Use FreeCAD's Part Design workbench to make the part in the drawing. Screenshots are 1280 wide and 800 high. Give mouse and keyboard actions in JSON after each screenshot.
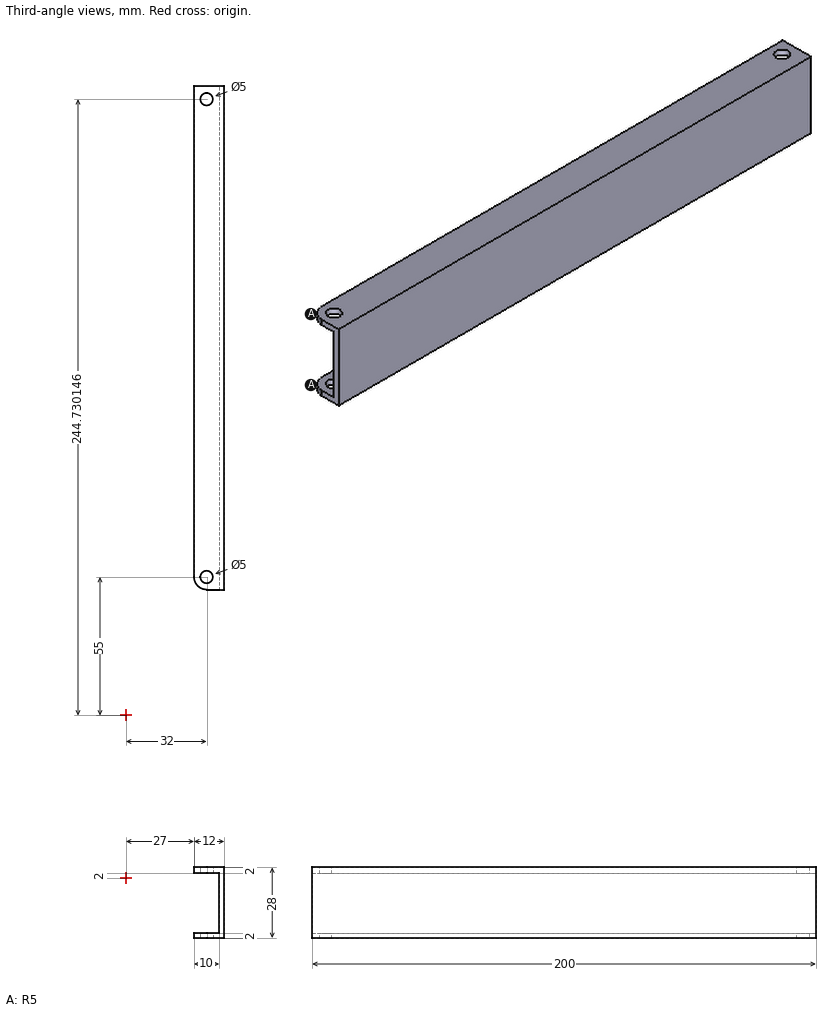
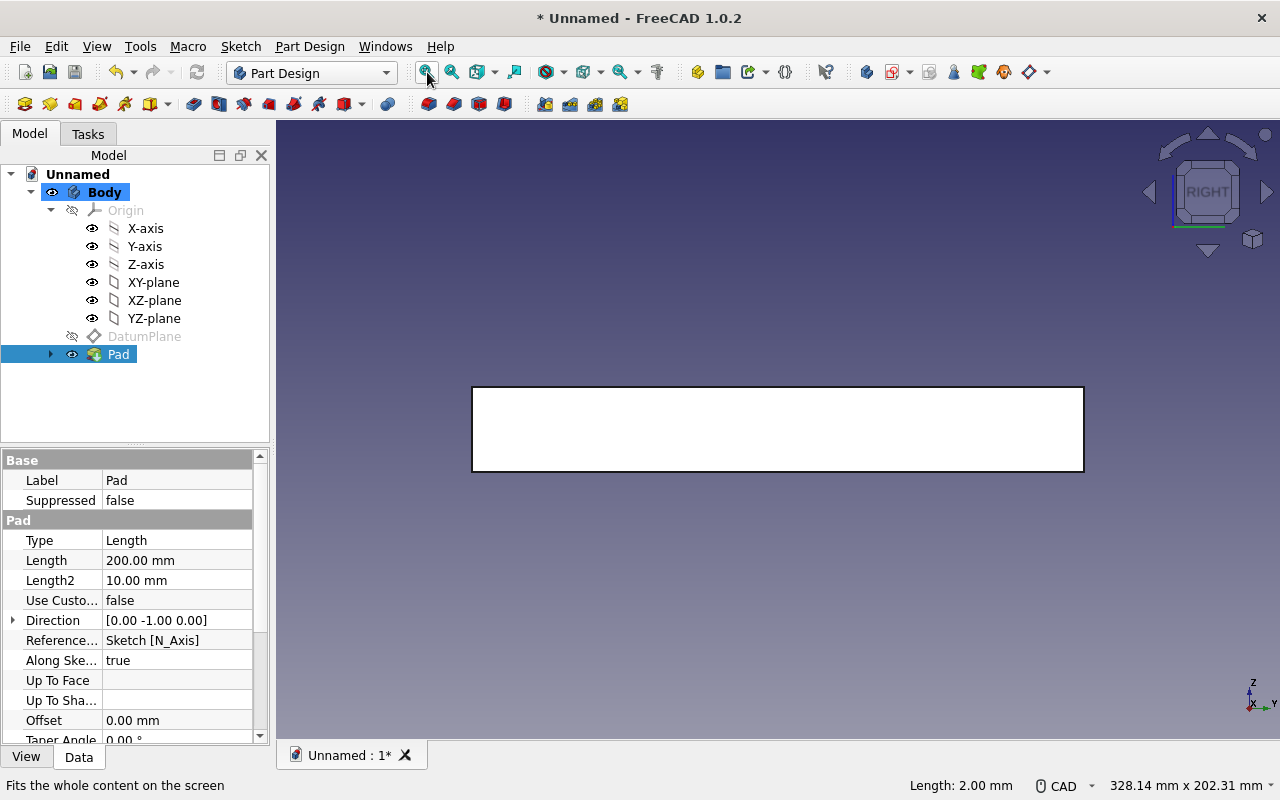
{"action": "key", "text": "5"}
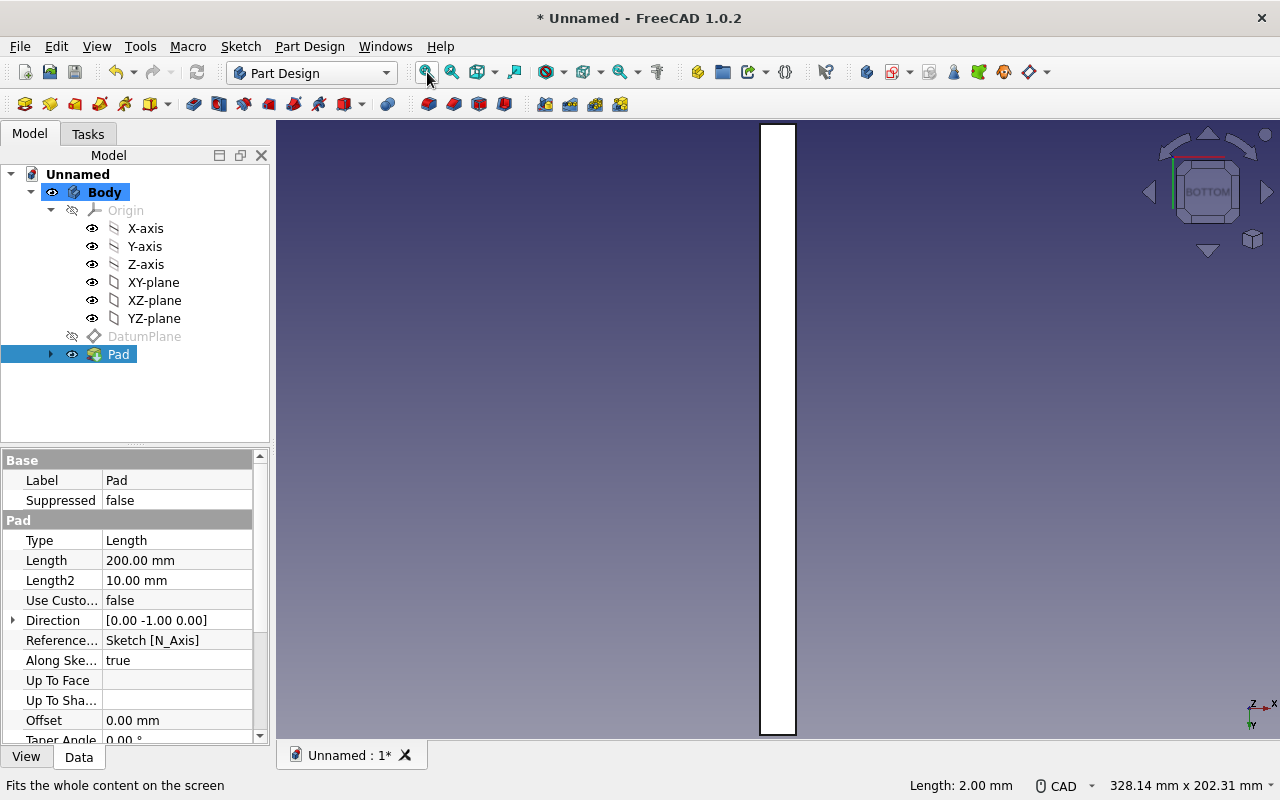
{"action": "key", "text": "4"}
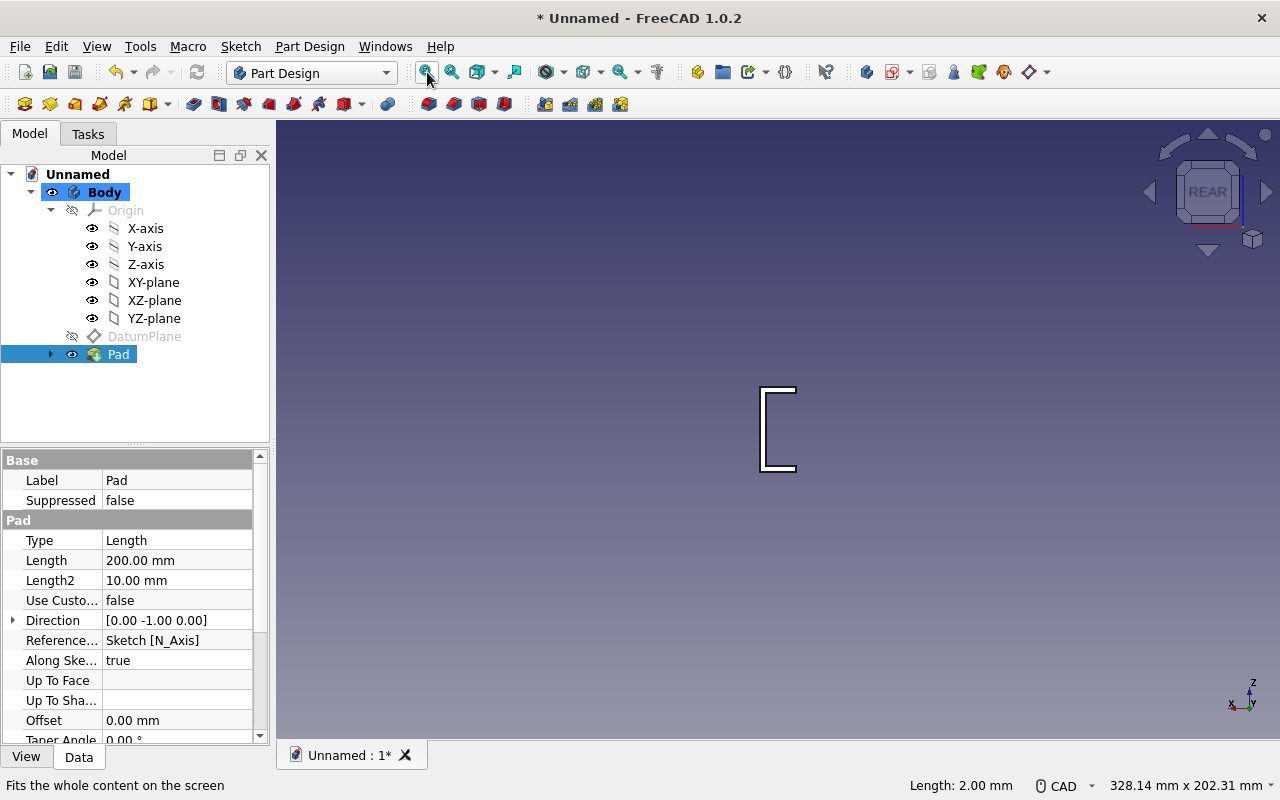
{"action": "left_click", "coordinate": [427, 72]}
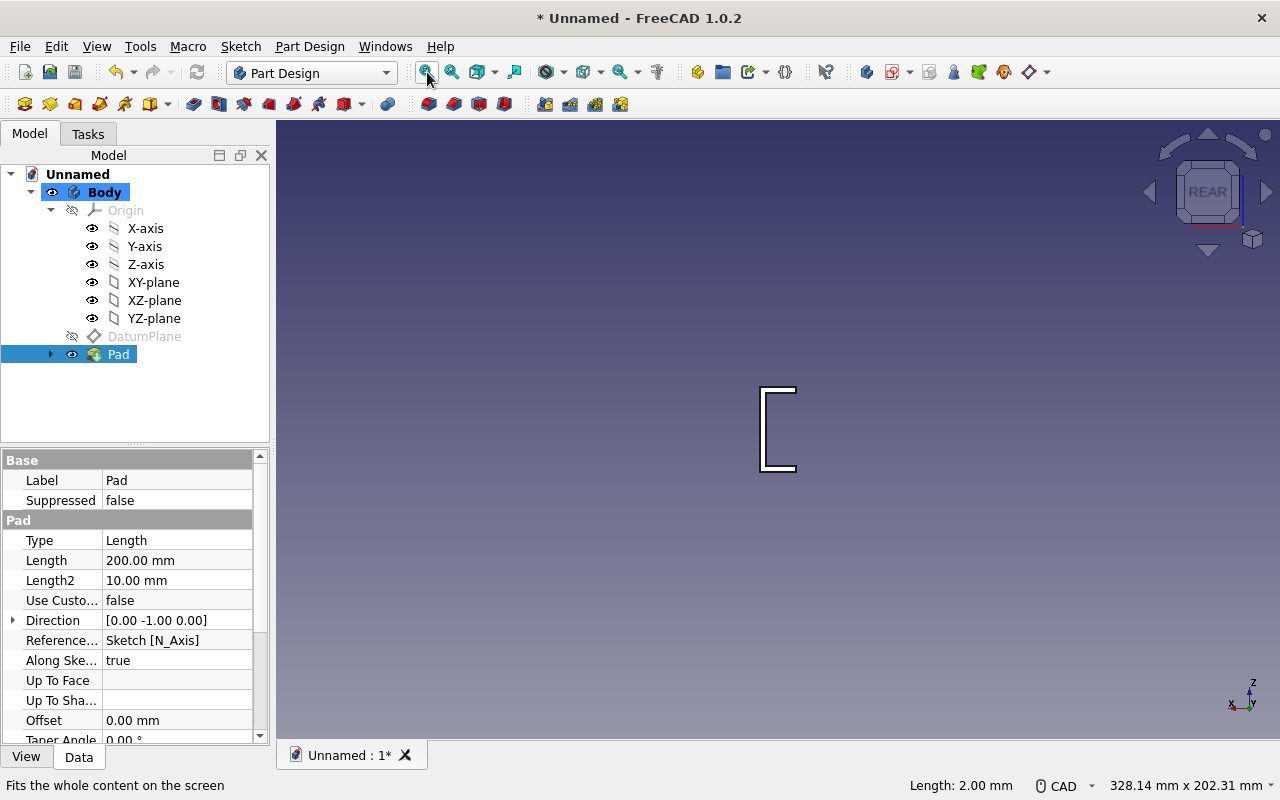
{"action": "scroll", "coordinate": [796, 468], "scroll_direction": "up", "scroll_amount": 10}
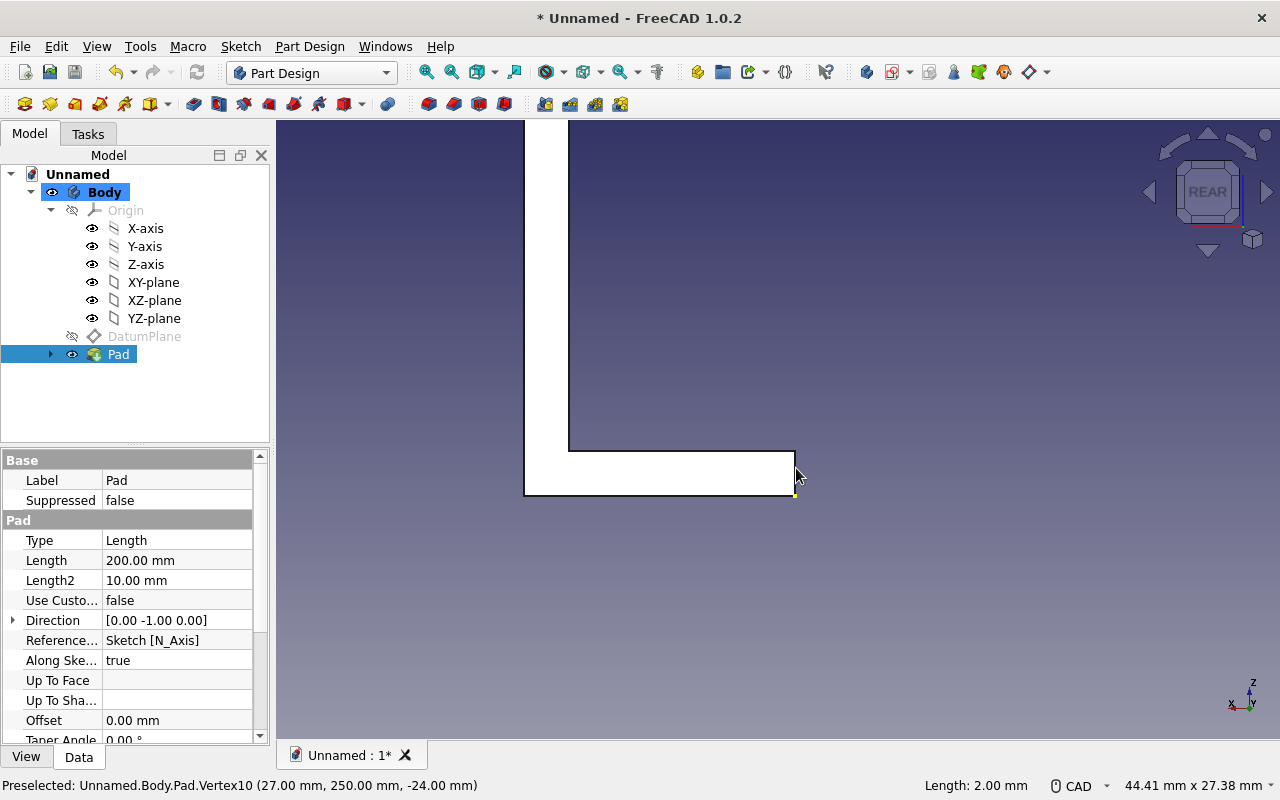
{"action": "left_click", "coordinate": [427, 72]}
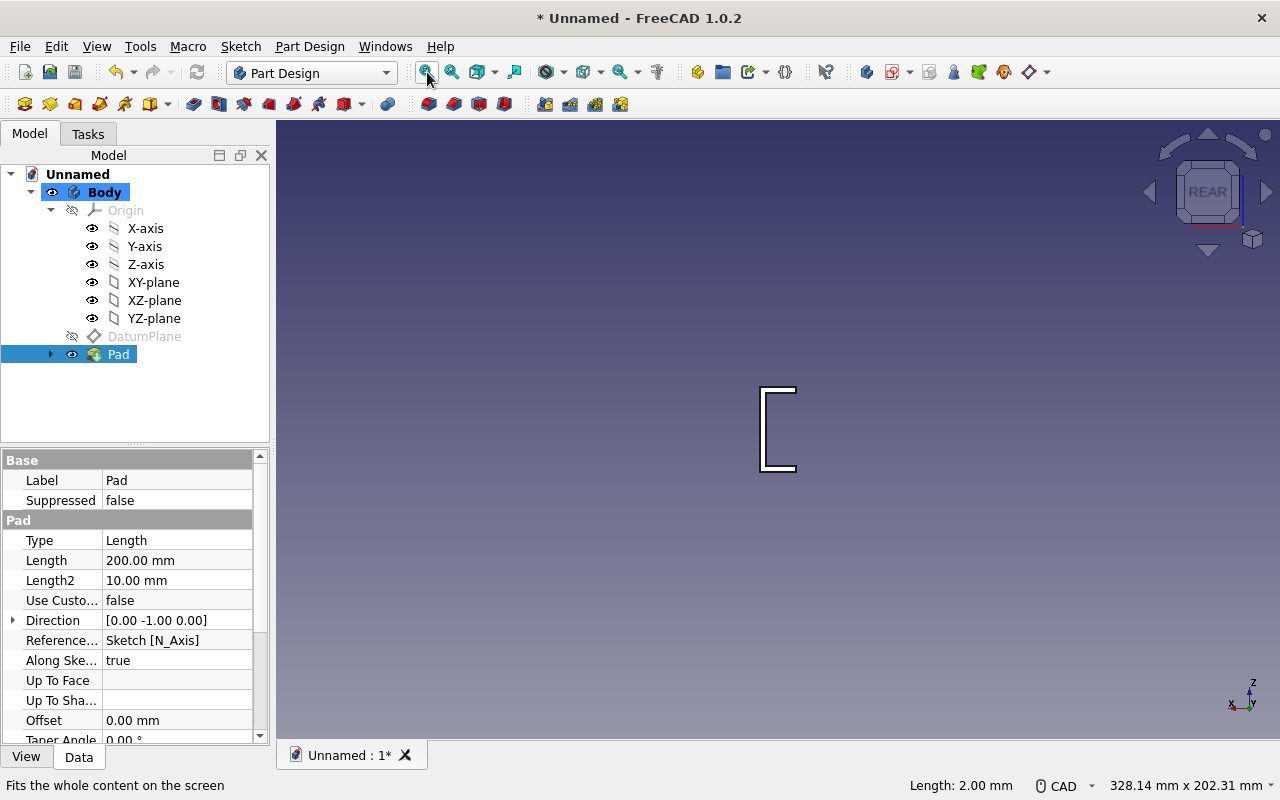
{"action": "key", "text": "6"}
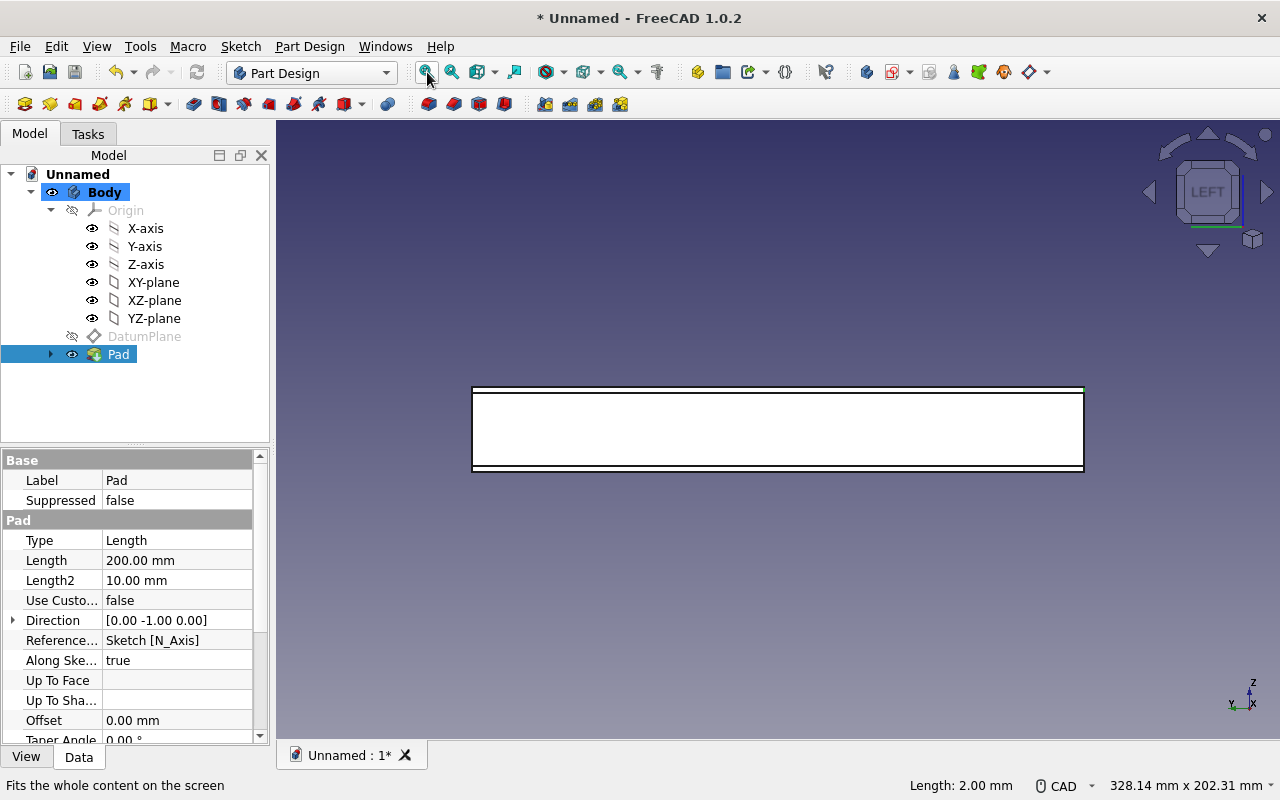
{"action": "scroll", "coordinate": [1084, 468], "scroll_direction": "up", "scroll_amount": 10}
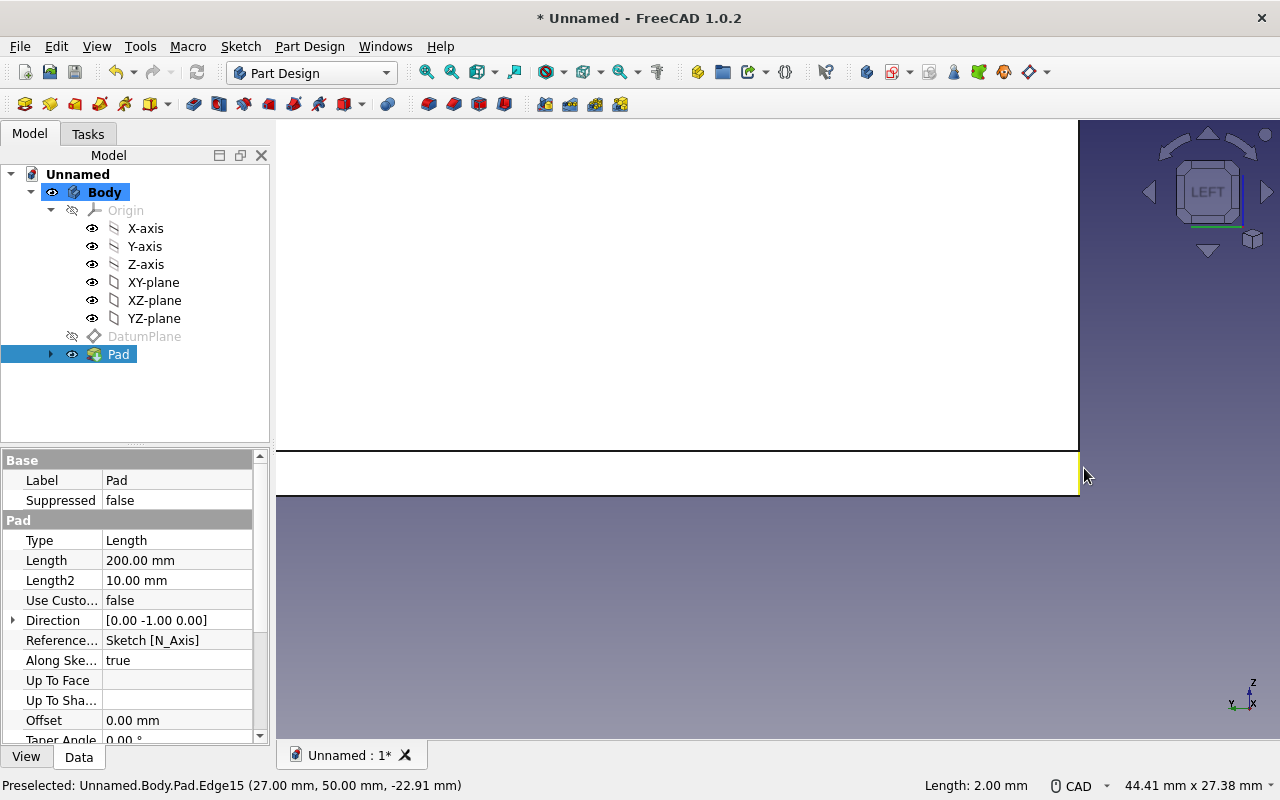
{"action": "left_click", "coordinate": [1079, 473], "text": "ctrl"}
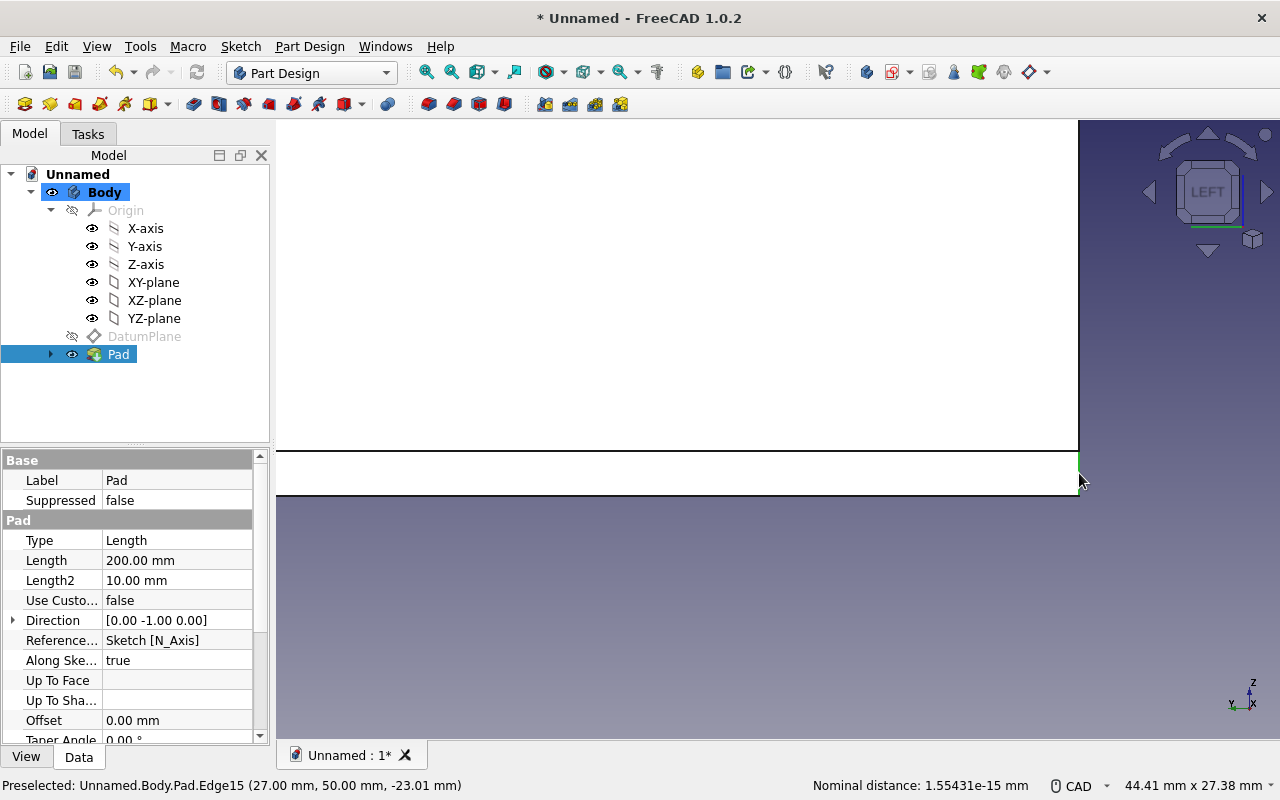
{"action": "left_click", "coordinate": [429, 104]}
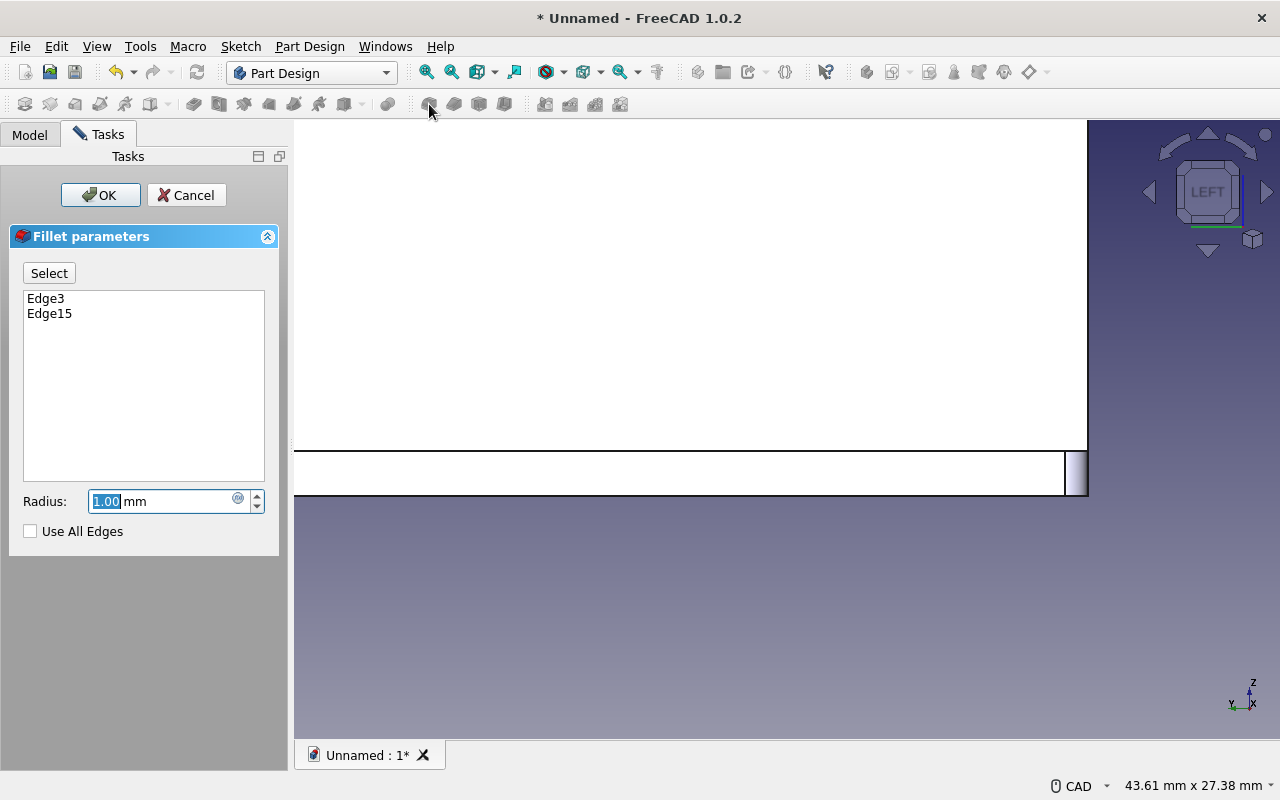
{"action": "type", "text": "5"}
{"action": "key", "text": "Tab"}